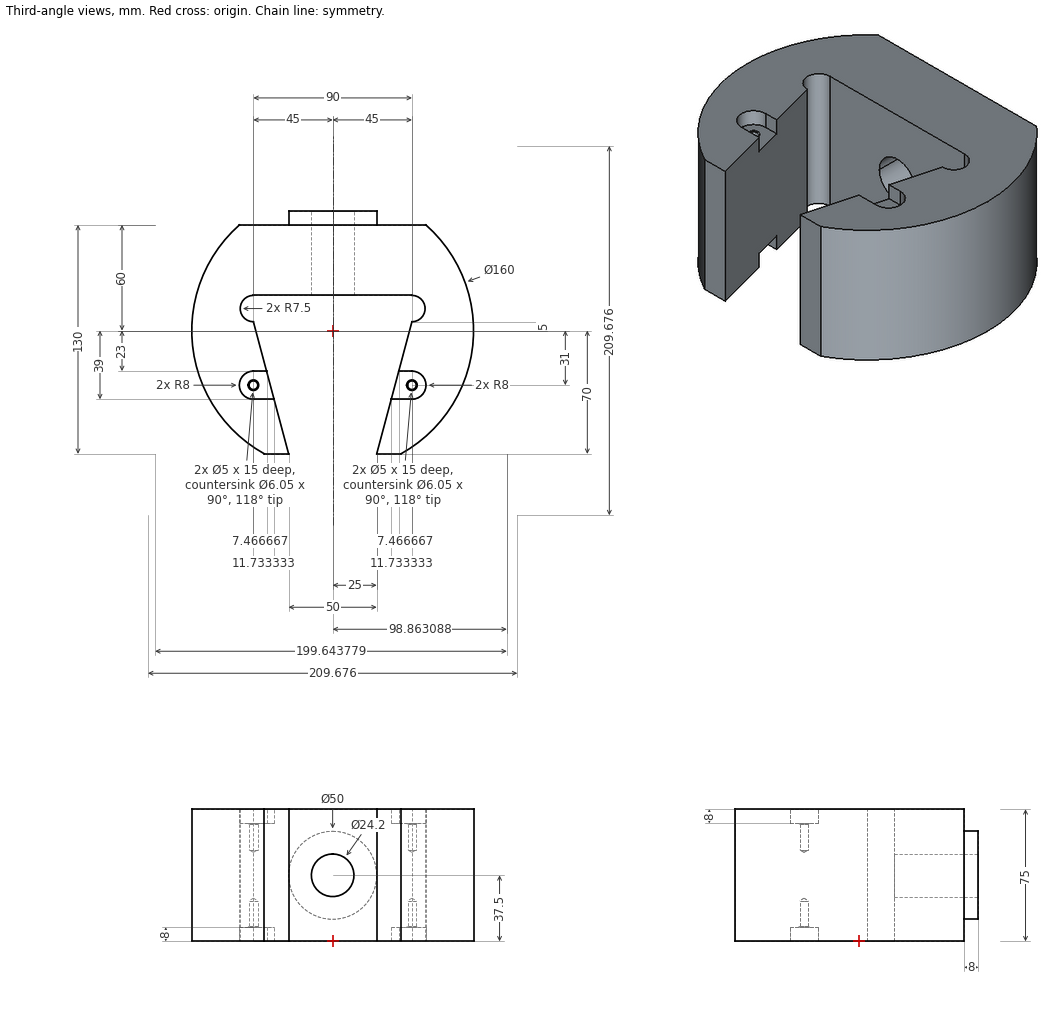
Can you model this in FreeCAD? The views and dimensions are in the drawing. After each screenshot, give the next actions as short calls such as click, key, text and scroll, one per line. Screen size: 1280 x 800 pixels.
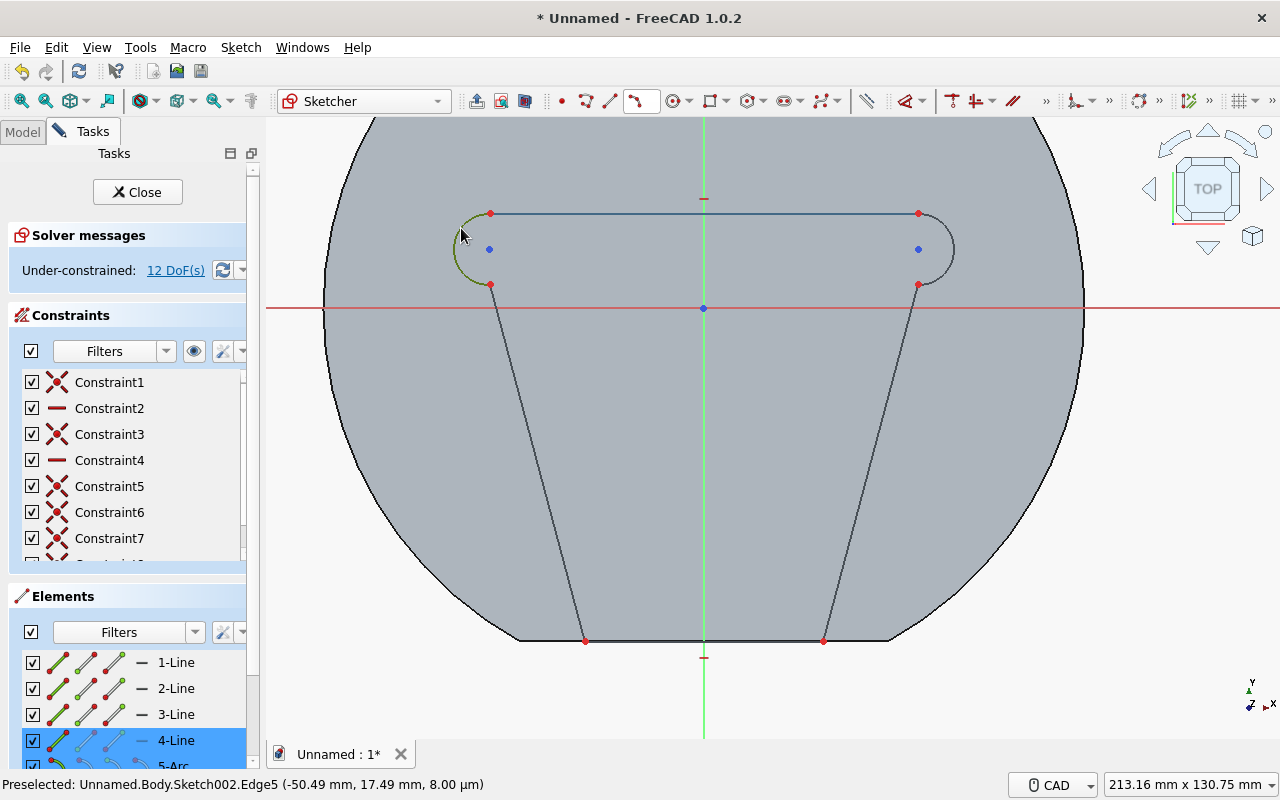
key(t)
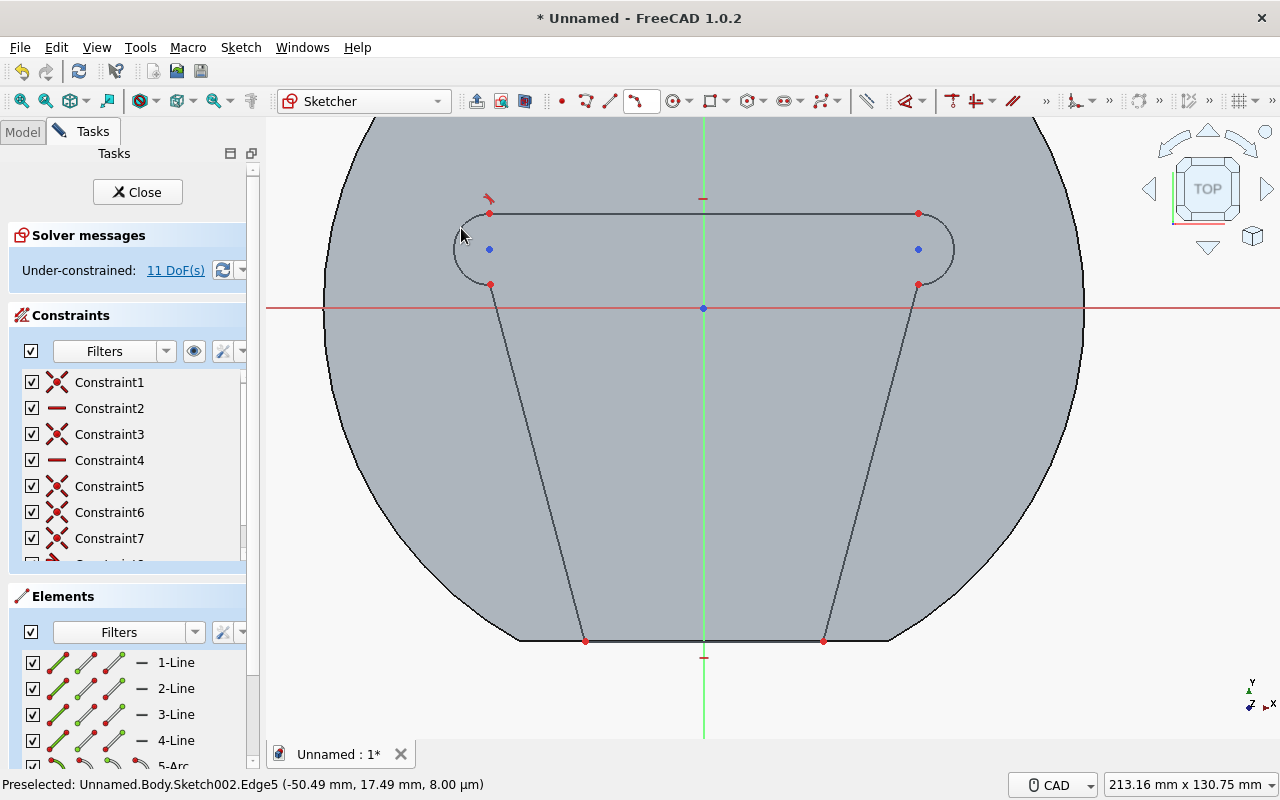
click(618, 214)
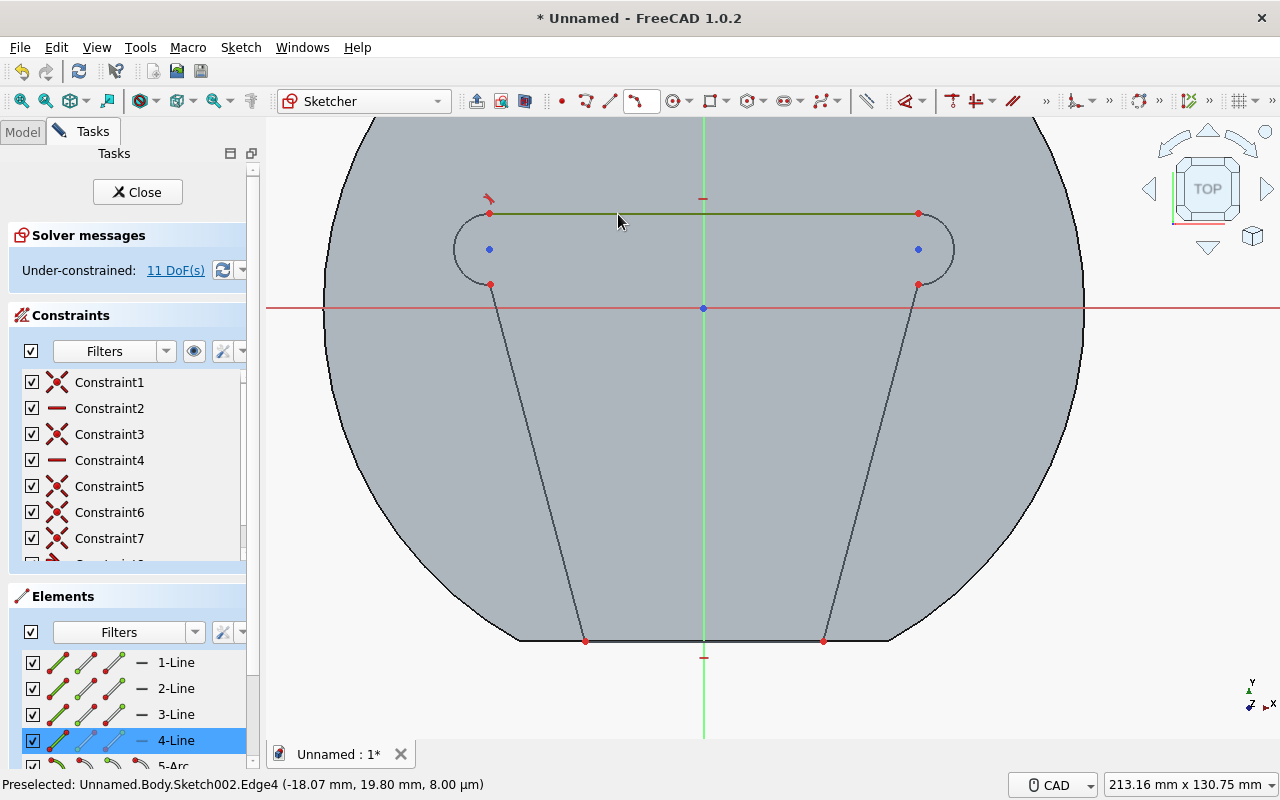
click(947, 271)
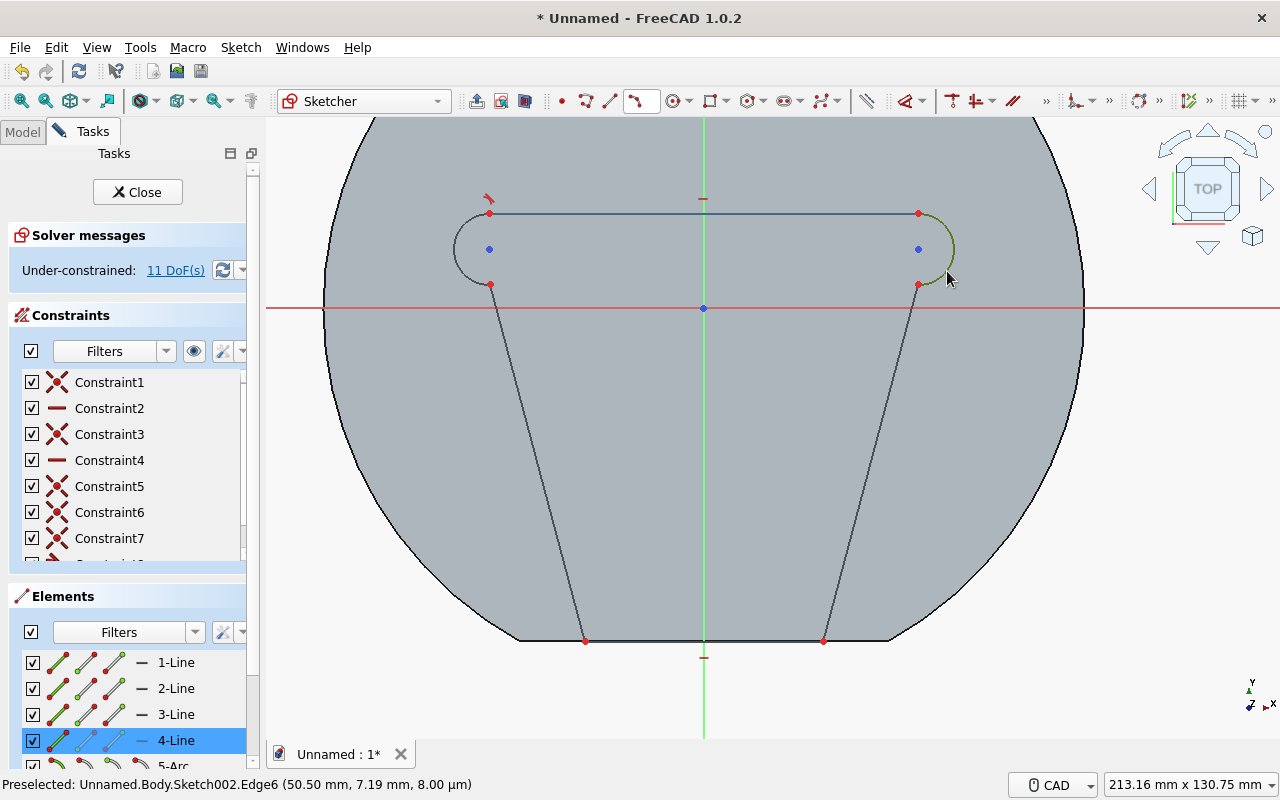
key(t)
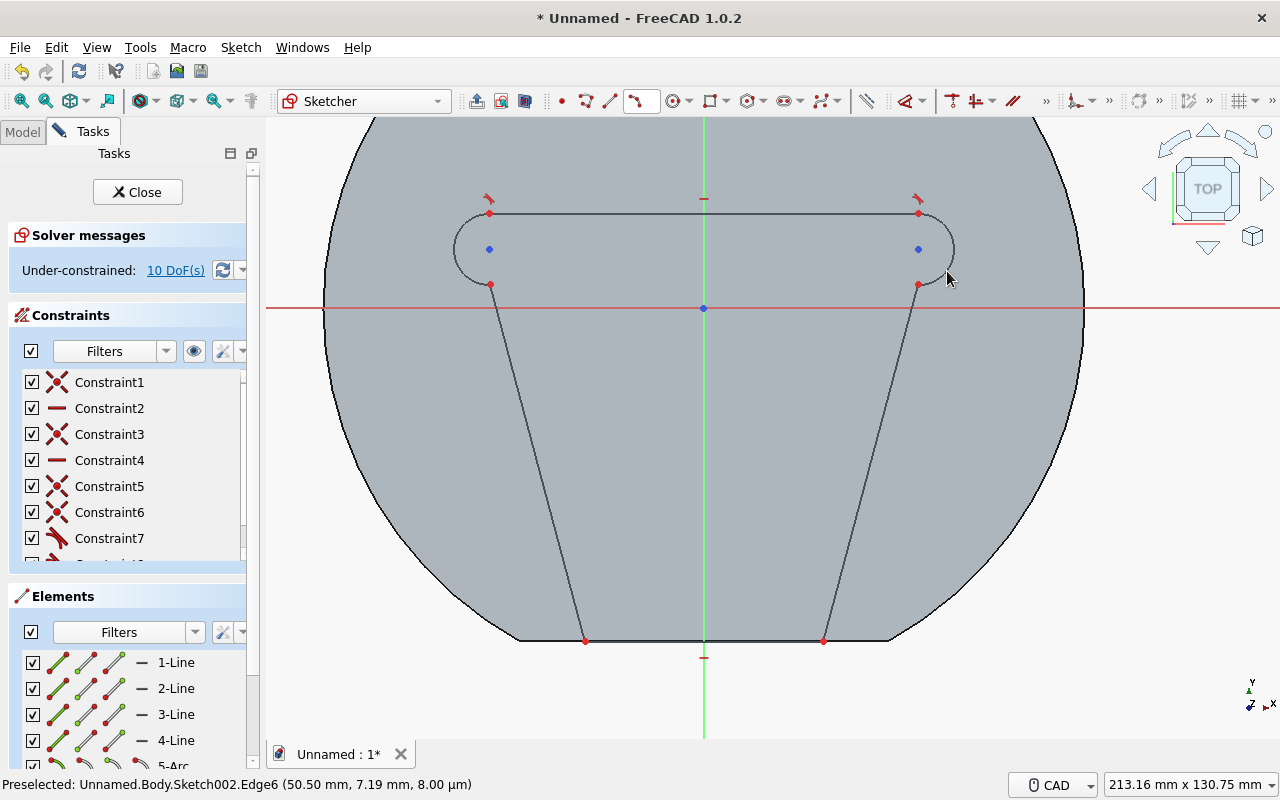
click(461, 229)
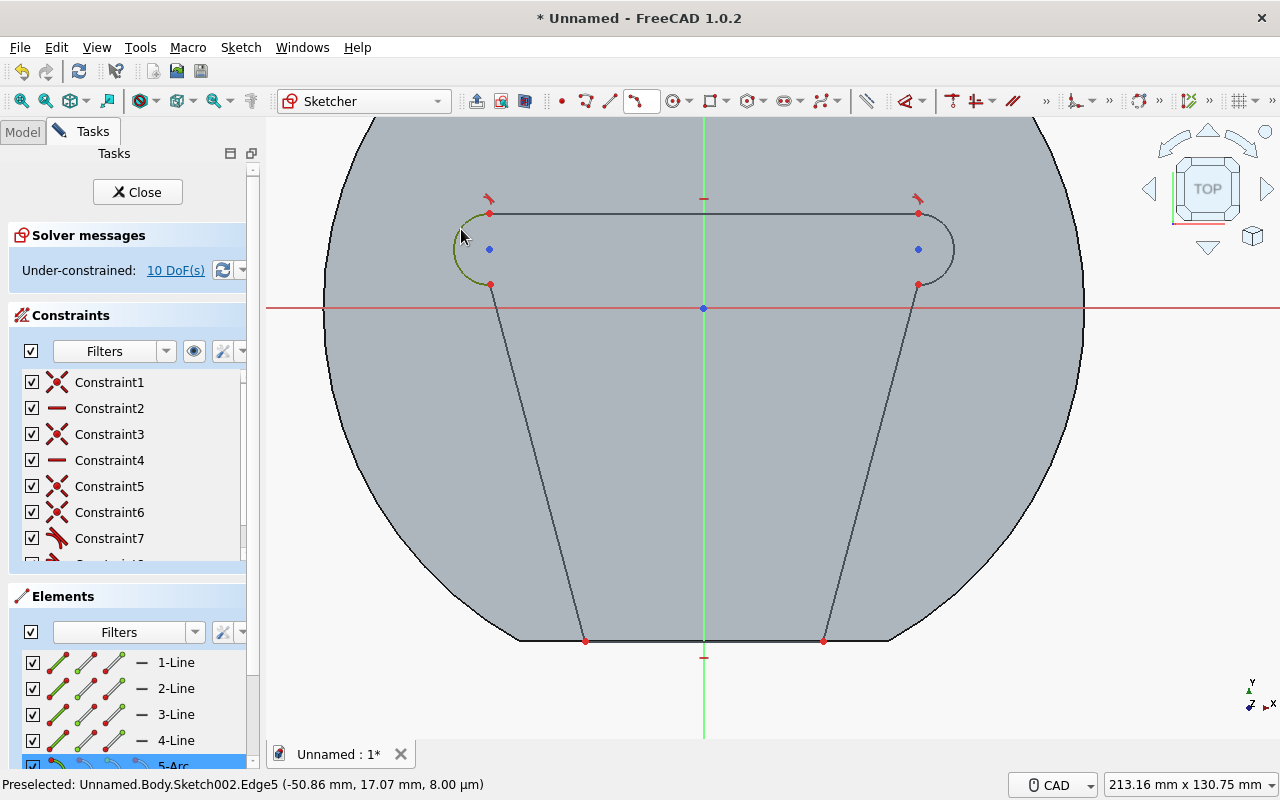
click(947, 271)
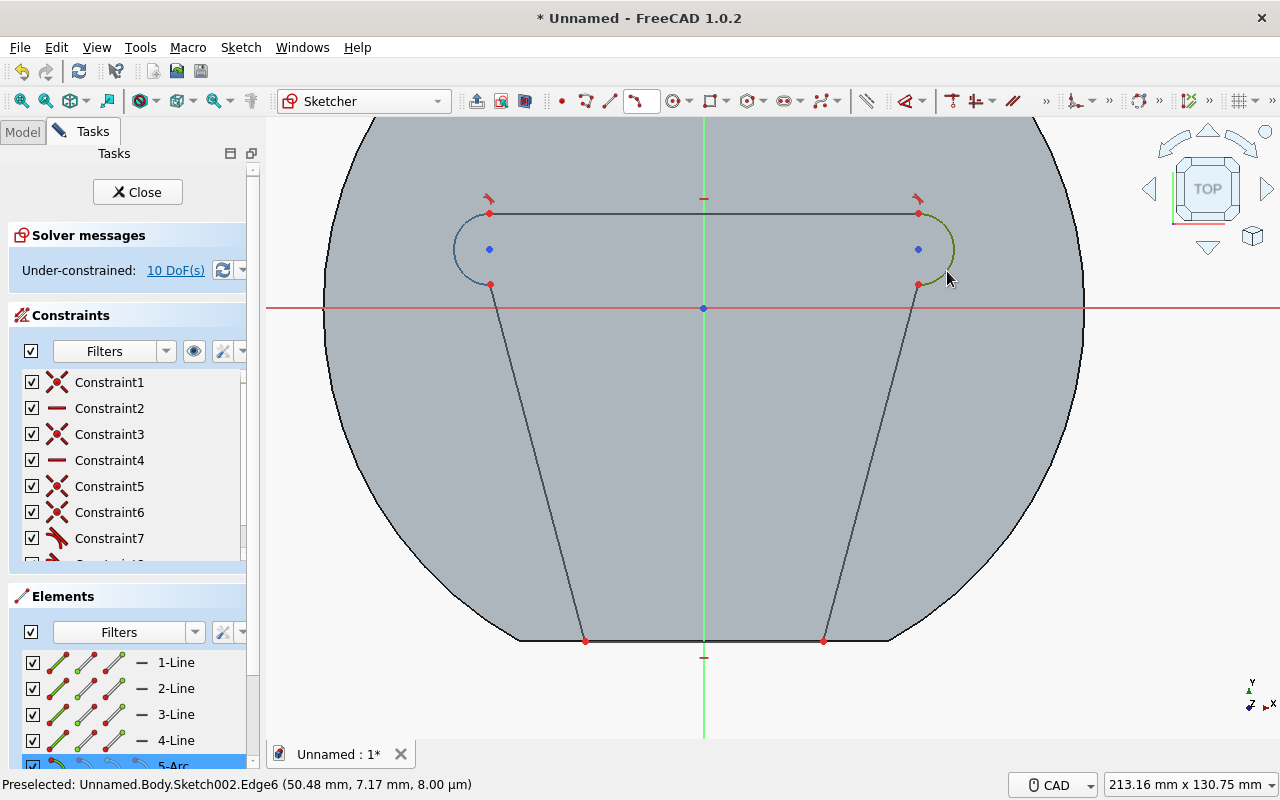
key(e)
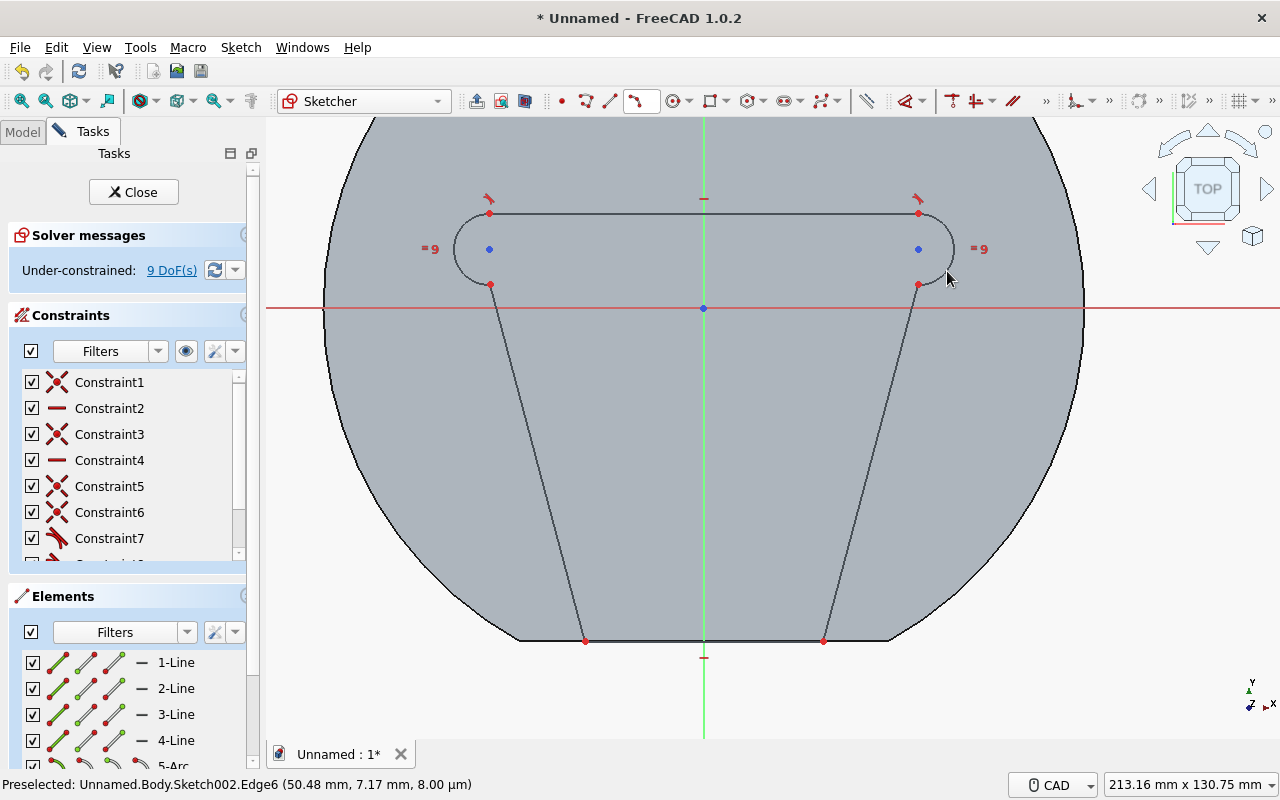
click(906, 102)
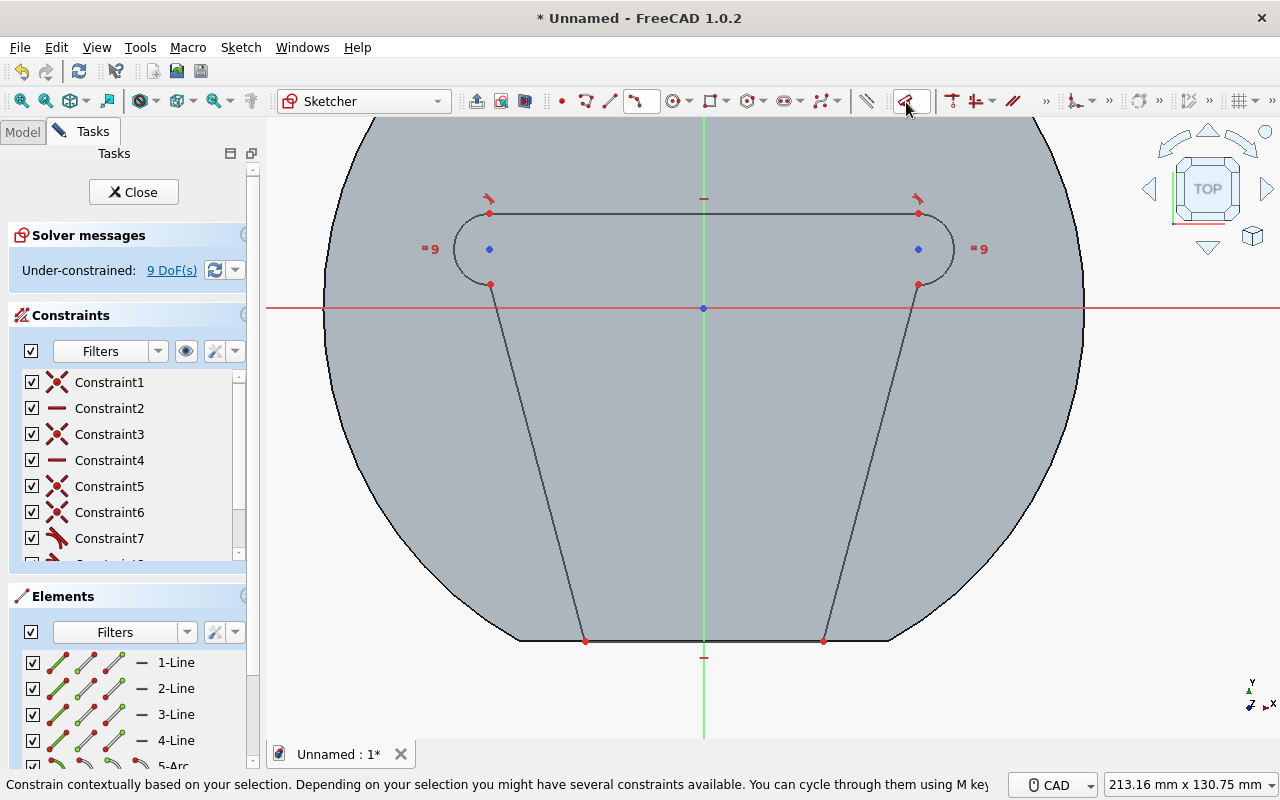
click(461, 229)
click(435, 210)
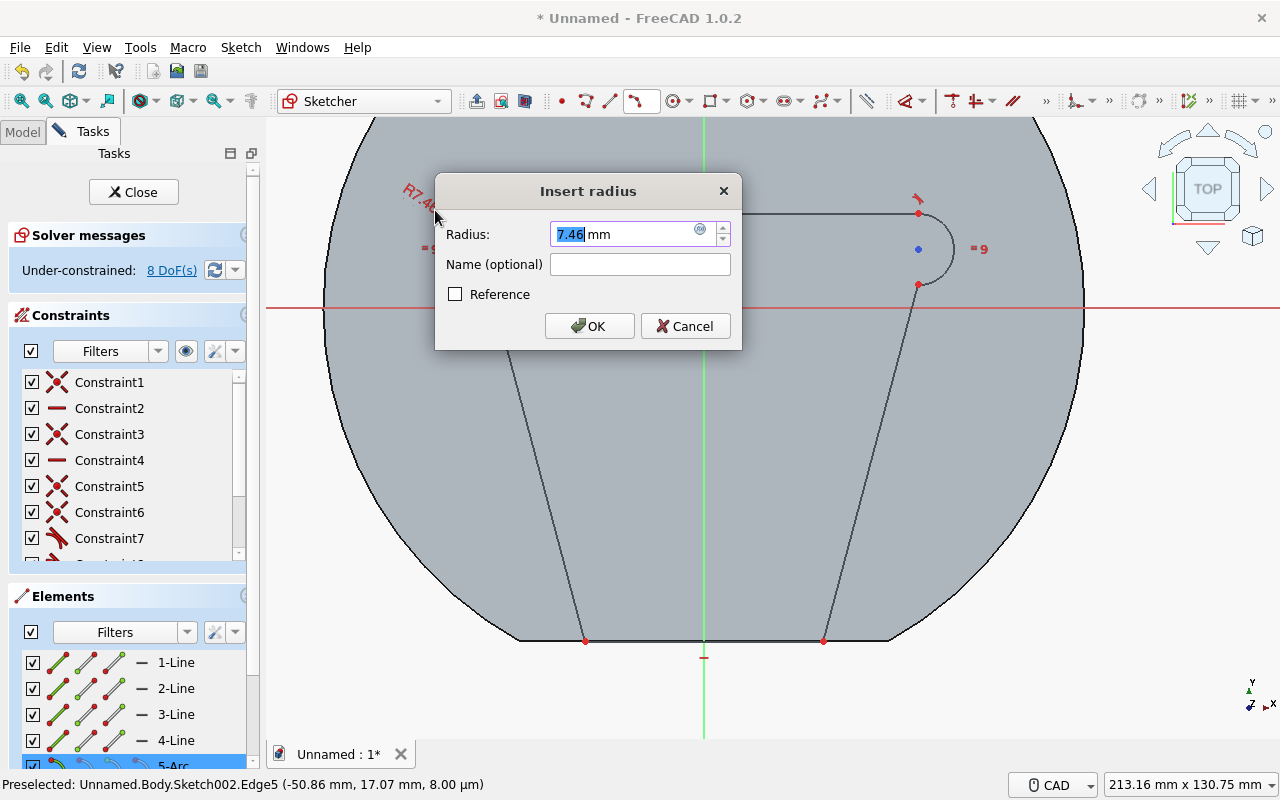
text(7.5)
key(Return)